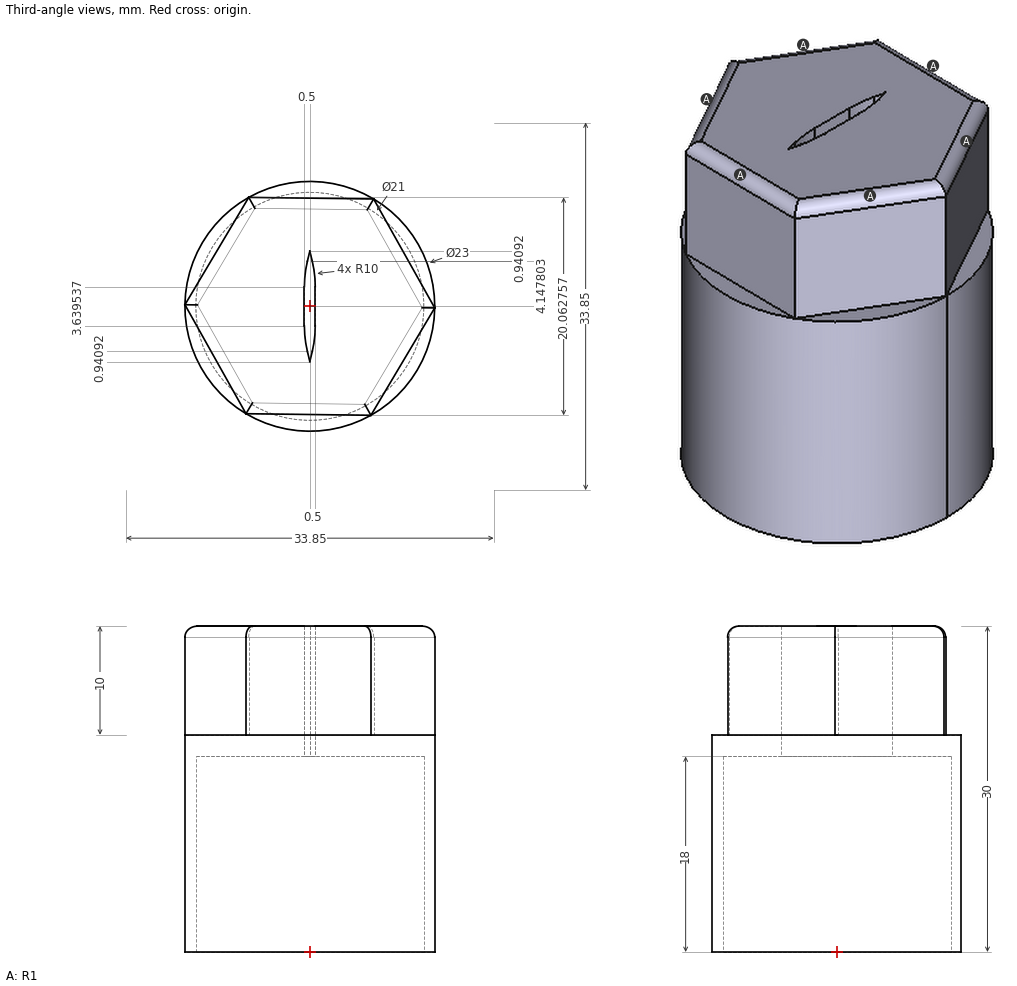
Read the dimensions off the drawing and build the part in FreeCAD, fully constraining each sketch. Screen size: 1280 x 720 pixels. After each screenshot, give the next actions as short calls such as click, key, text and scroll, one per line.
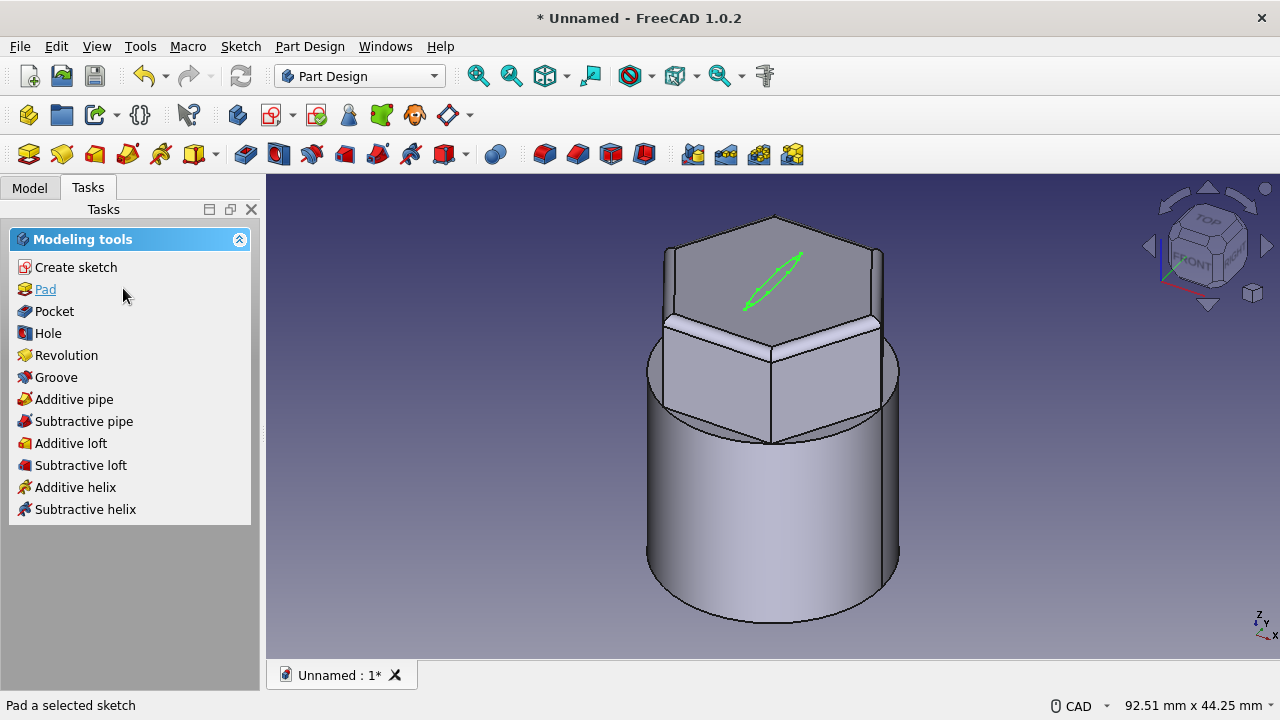
click(246, 154)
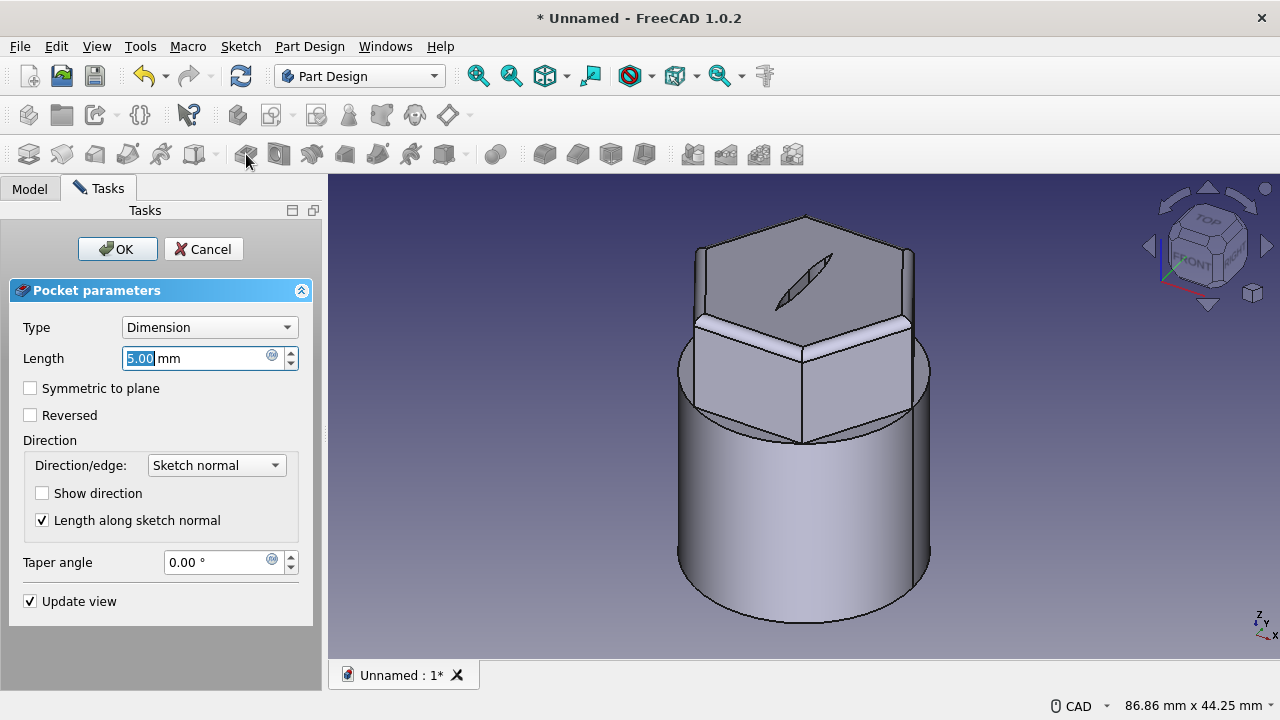
click(210, 328)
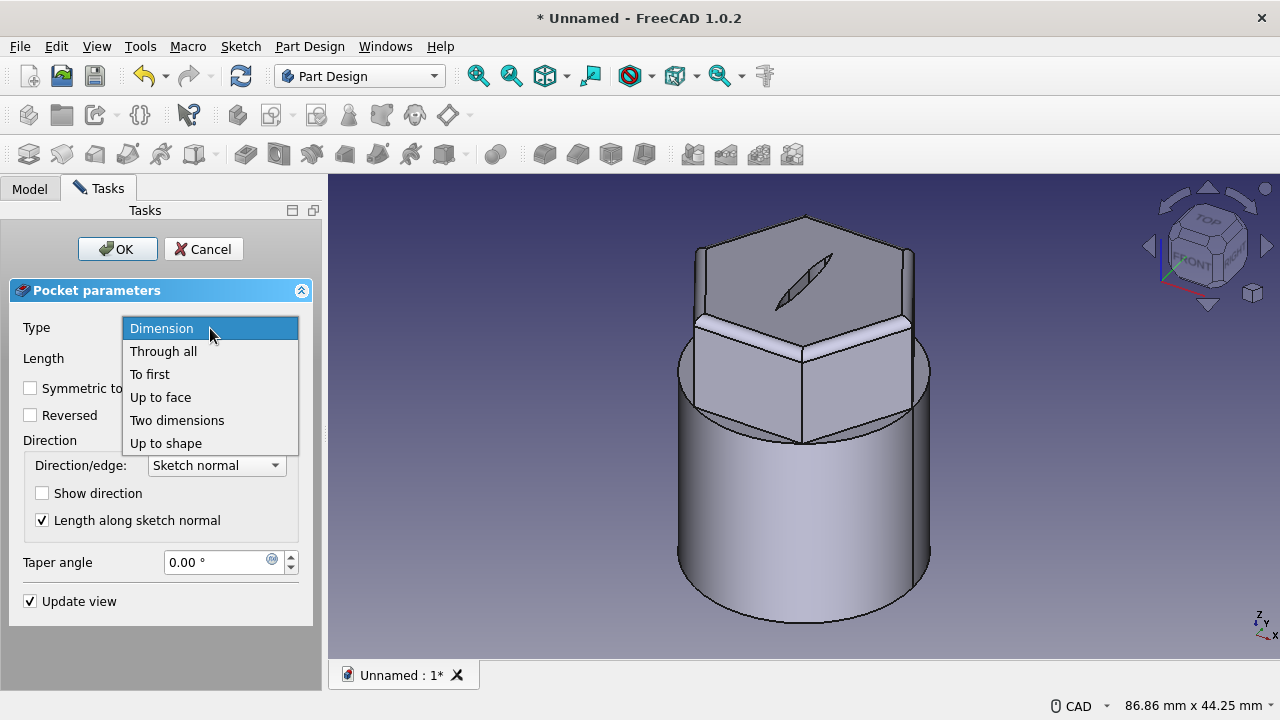
click(208, 352)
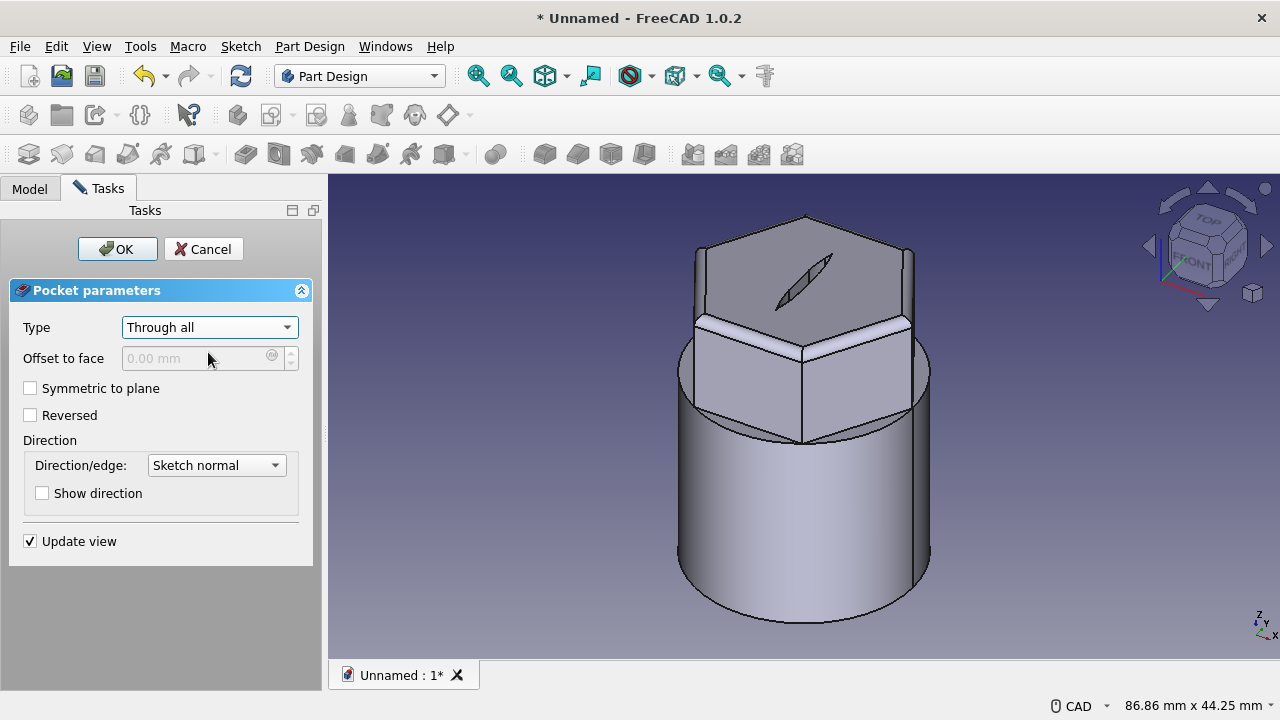
click(118, 249)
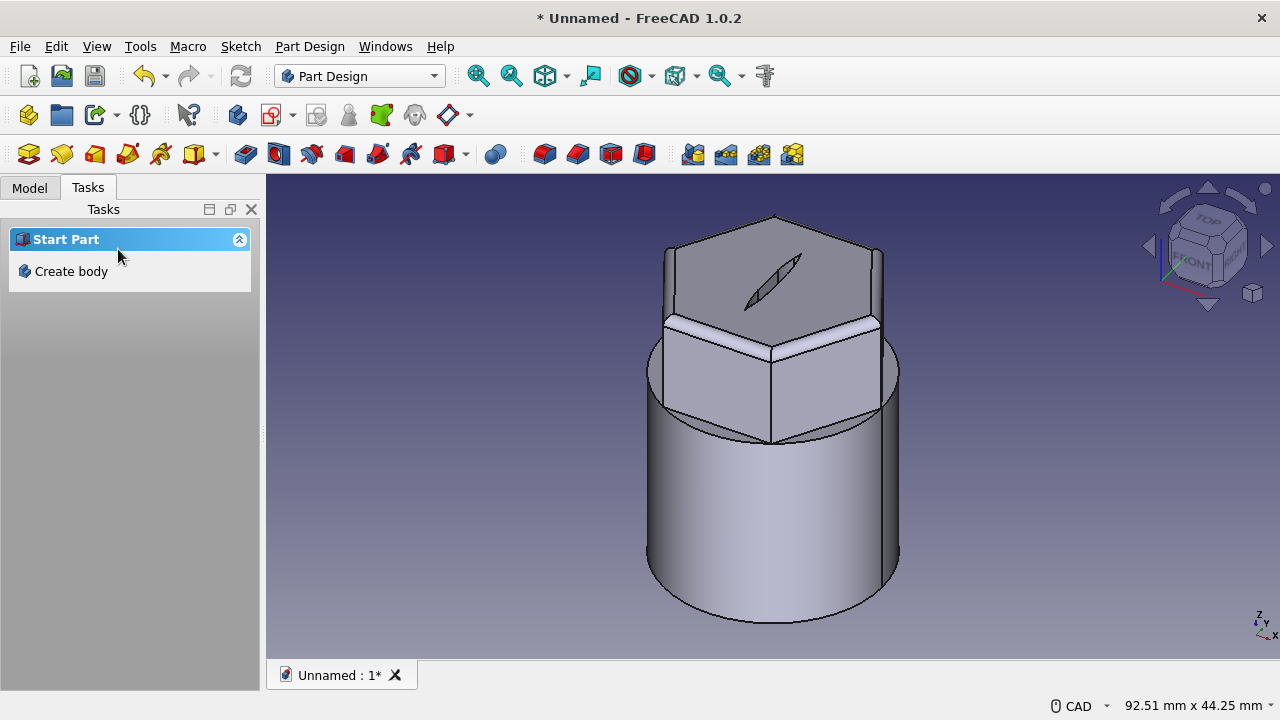
key(5)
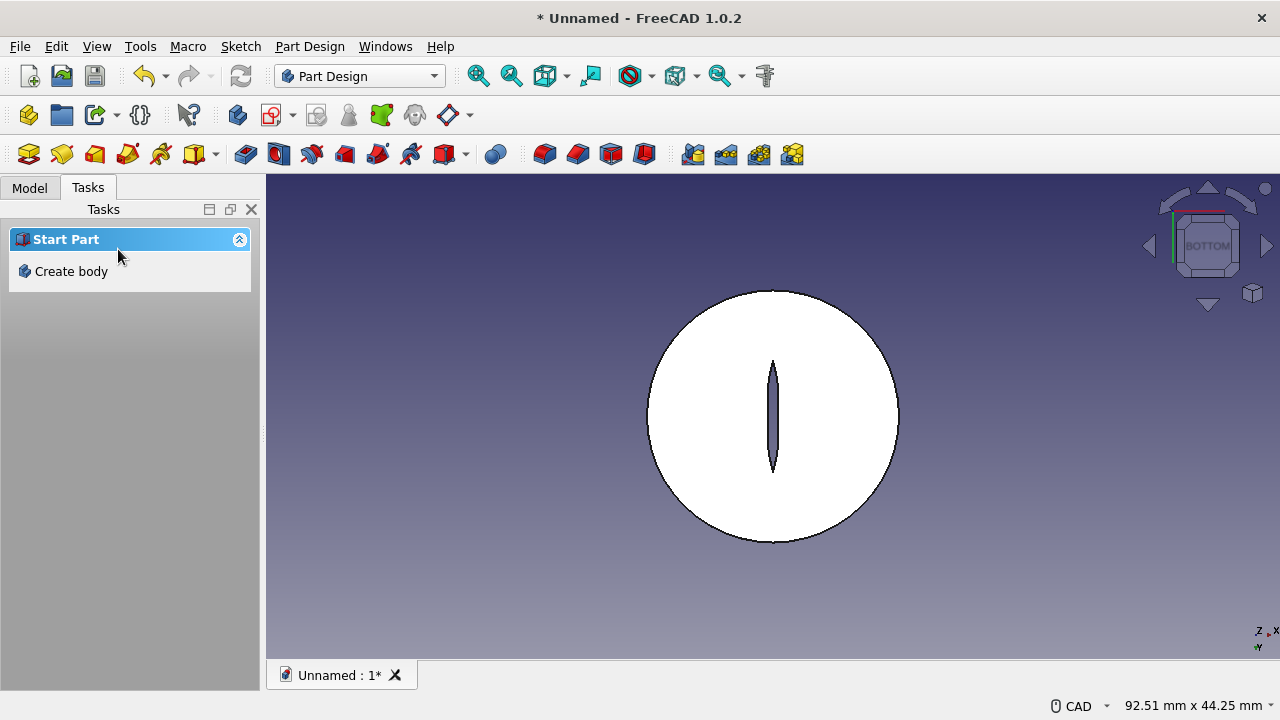
click(845, 415)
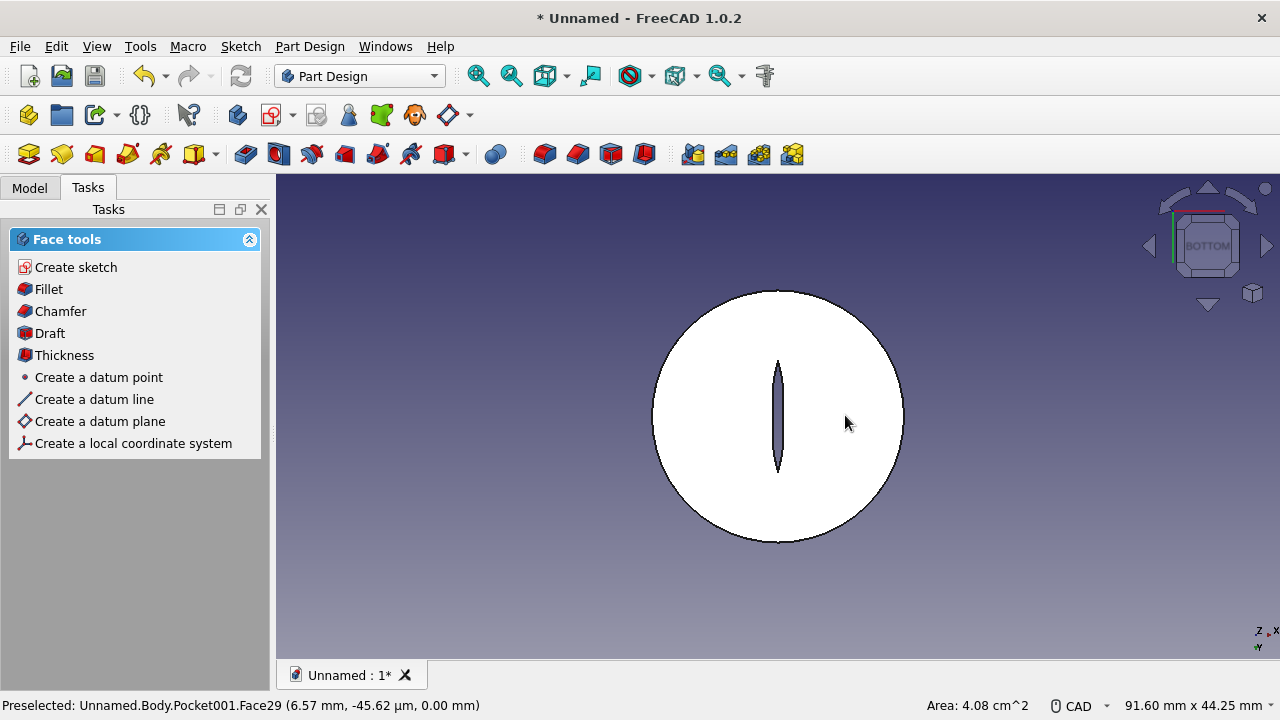
click(270, 116)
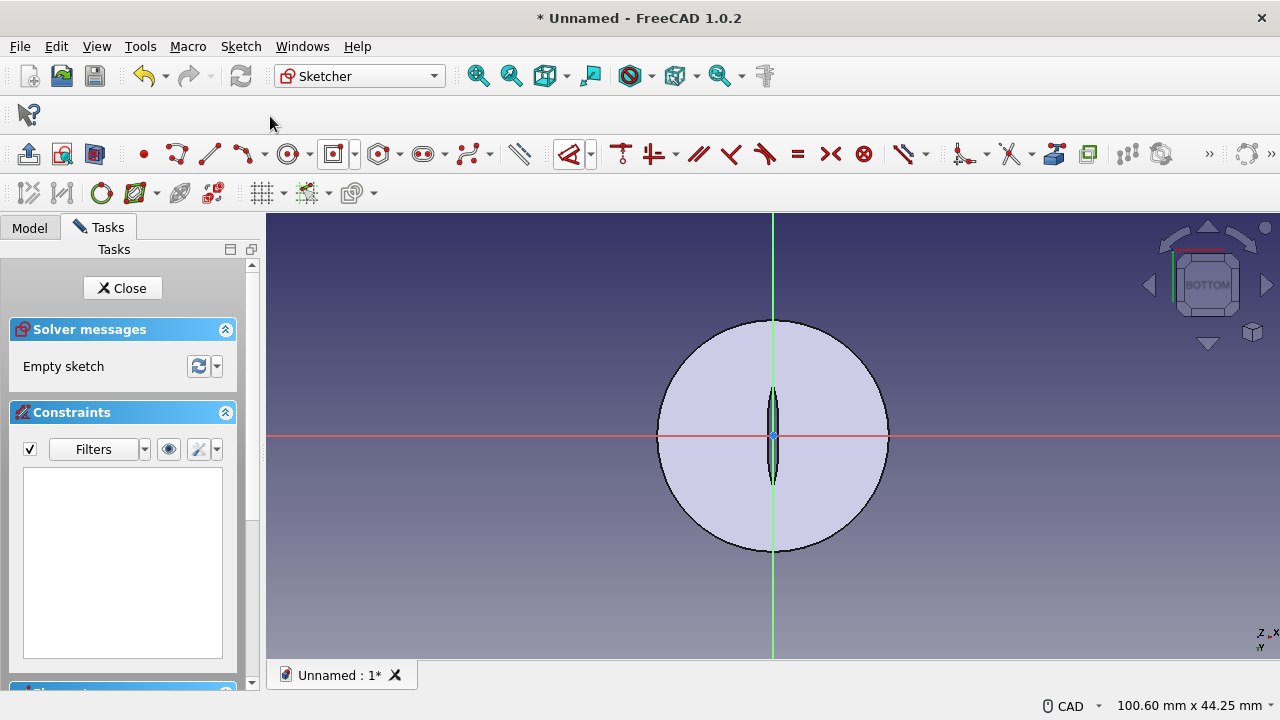
click(288, 154)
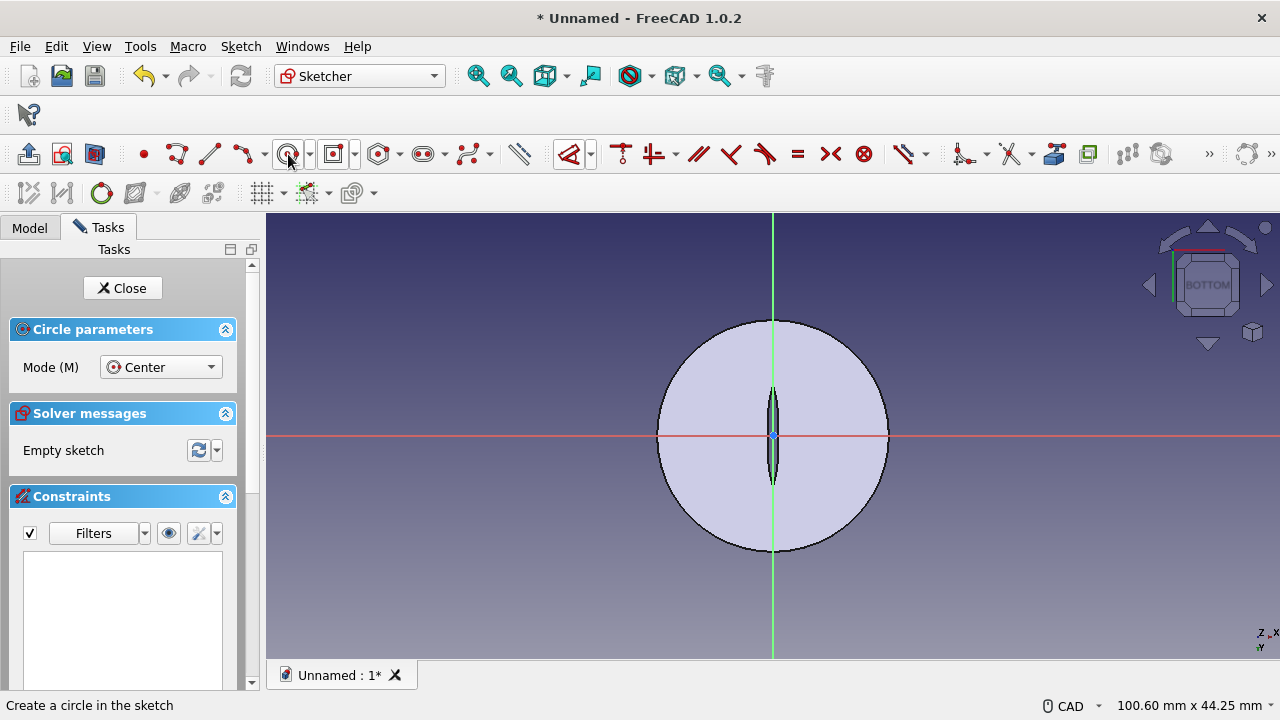
click(773, 436)
click(848, 361)
key(Escape)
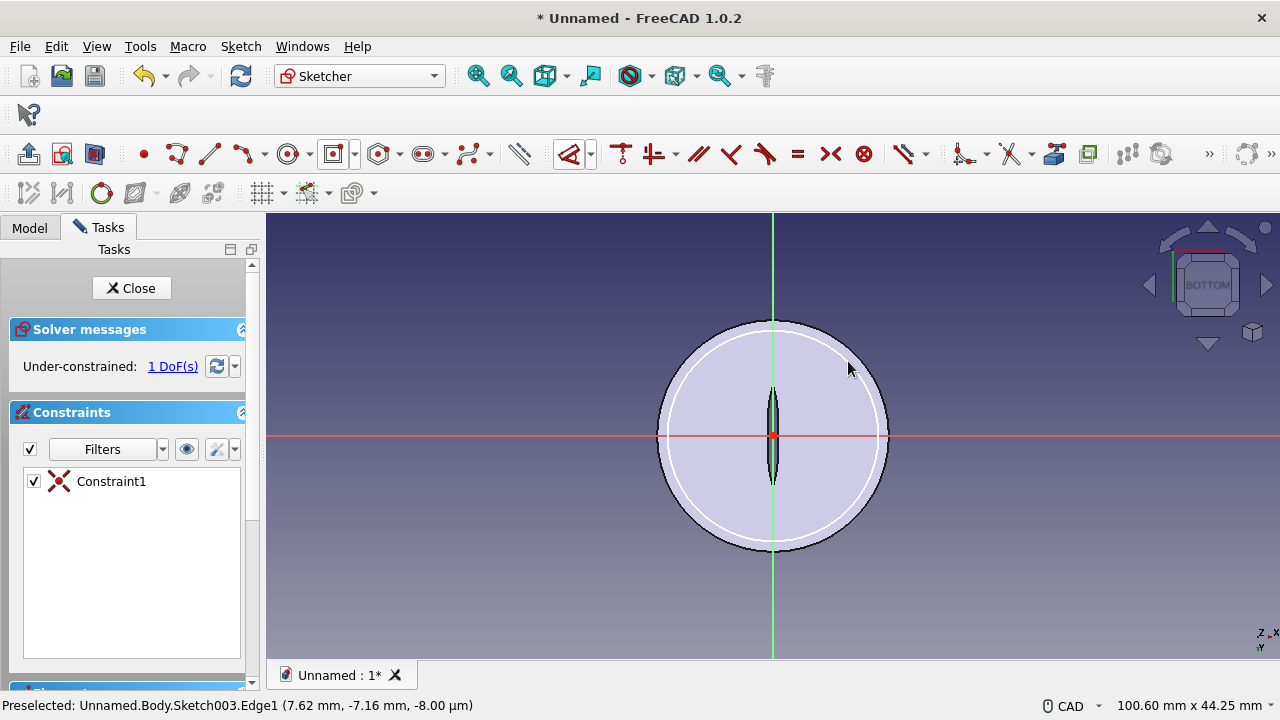
click(847, 361)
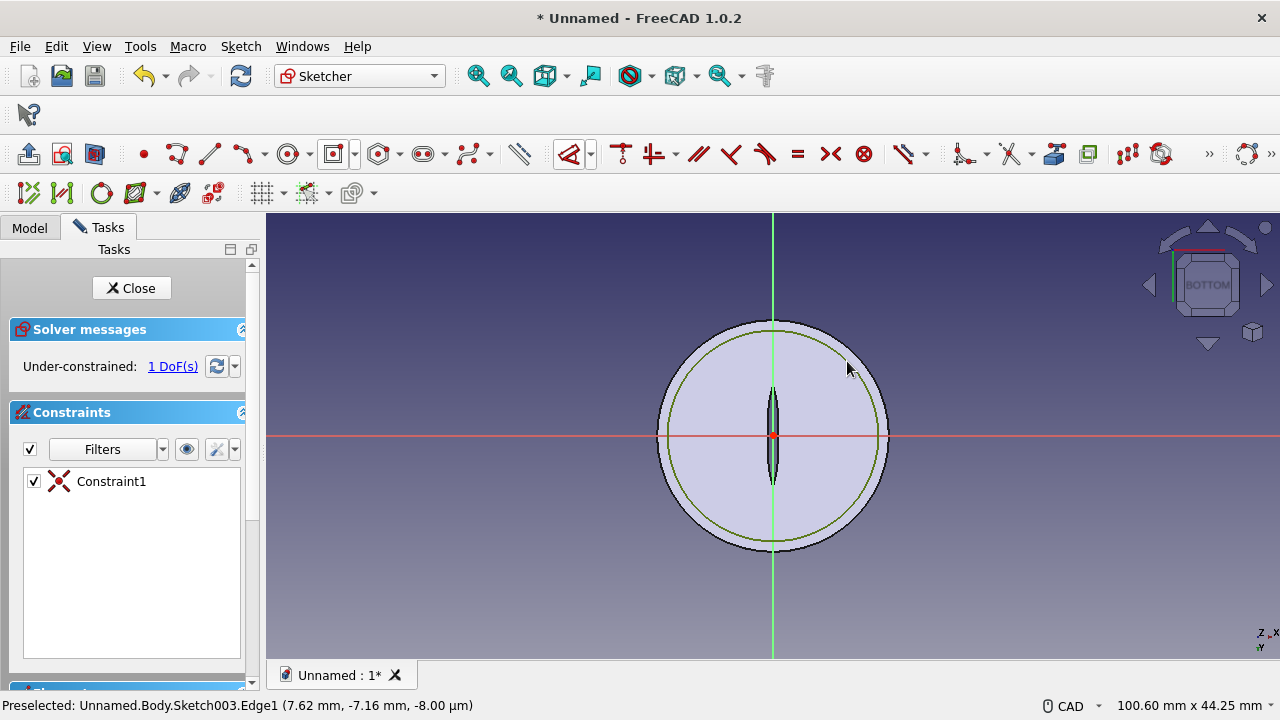
click(590, 154)